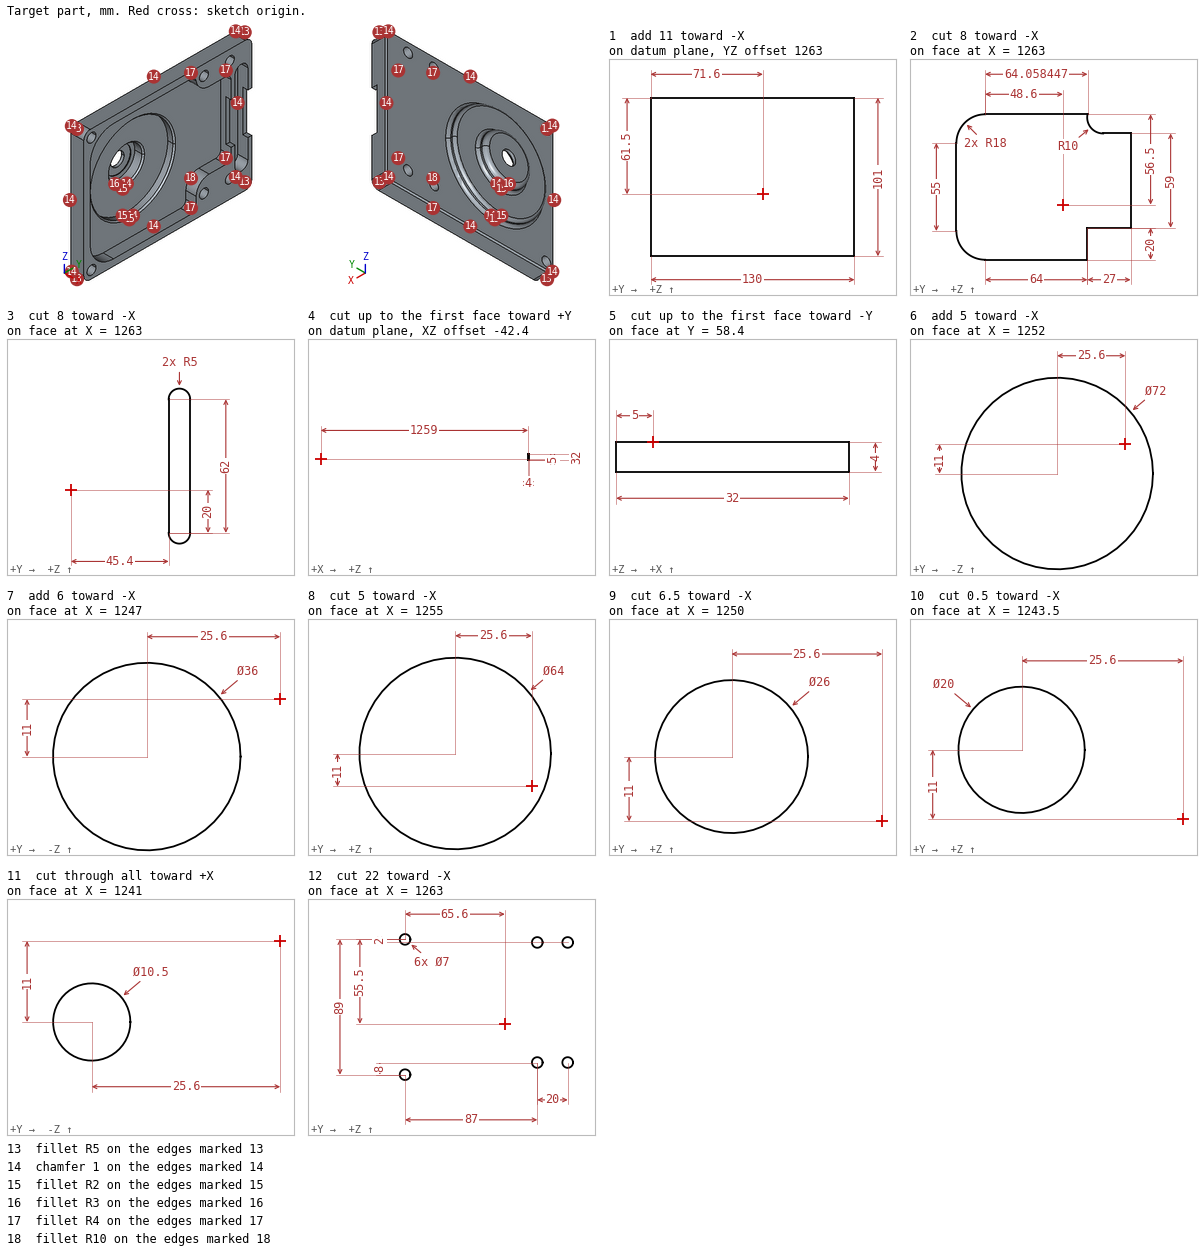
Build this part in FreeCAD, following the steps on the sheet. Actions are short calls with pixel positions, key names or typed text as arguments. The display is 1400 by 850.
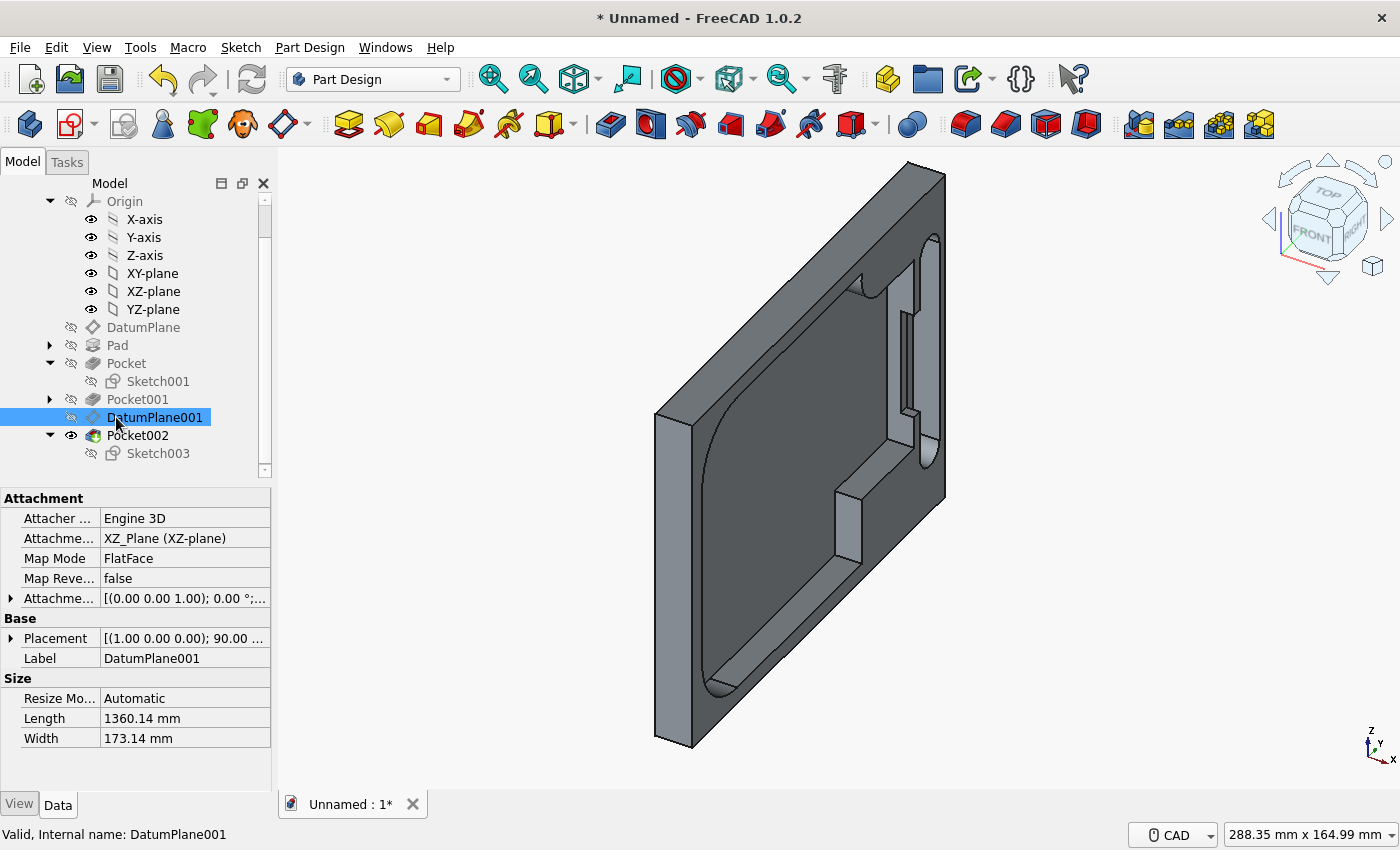
key(4)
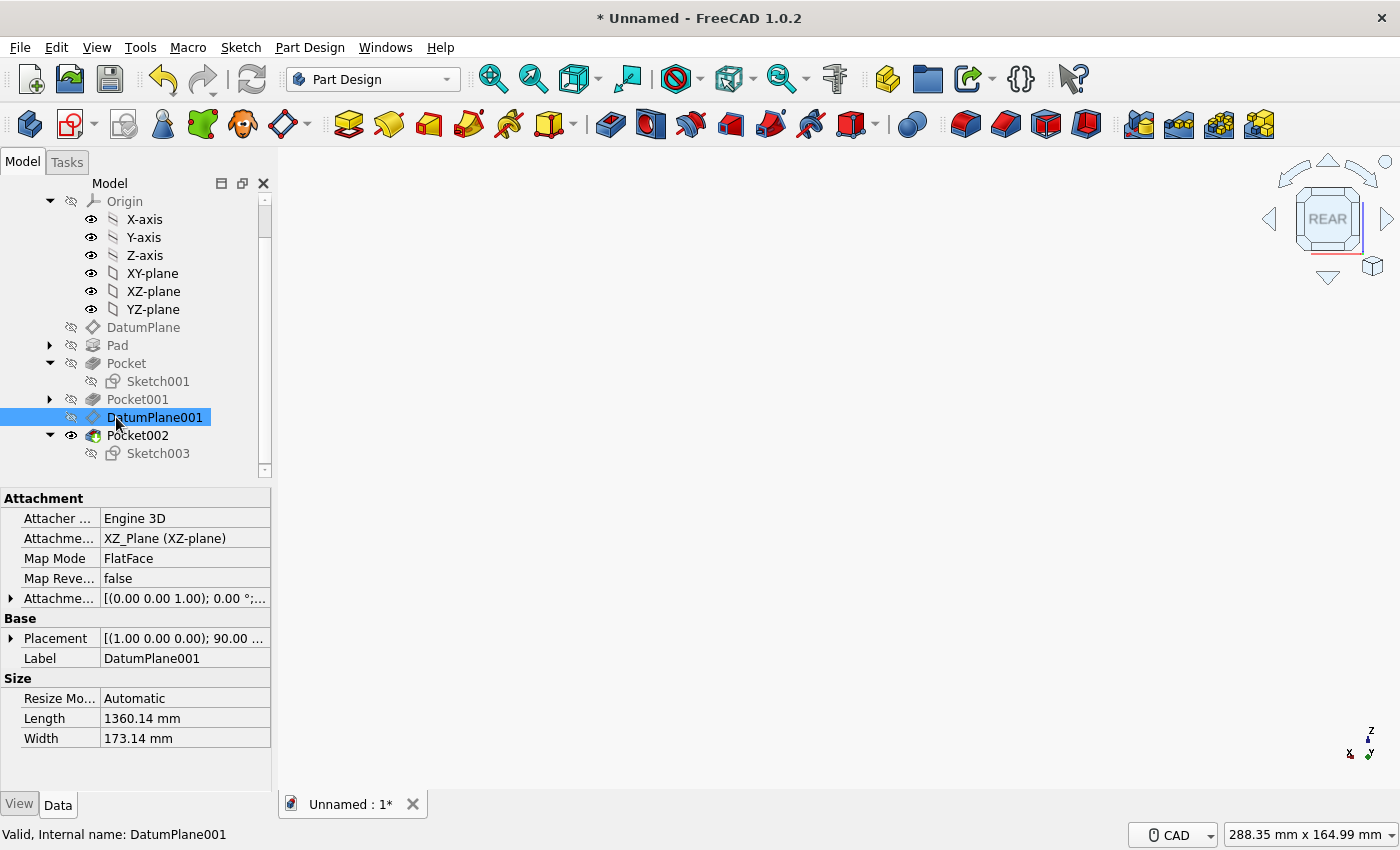
key(v)
key(f)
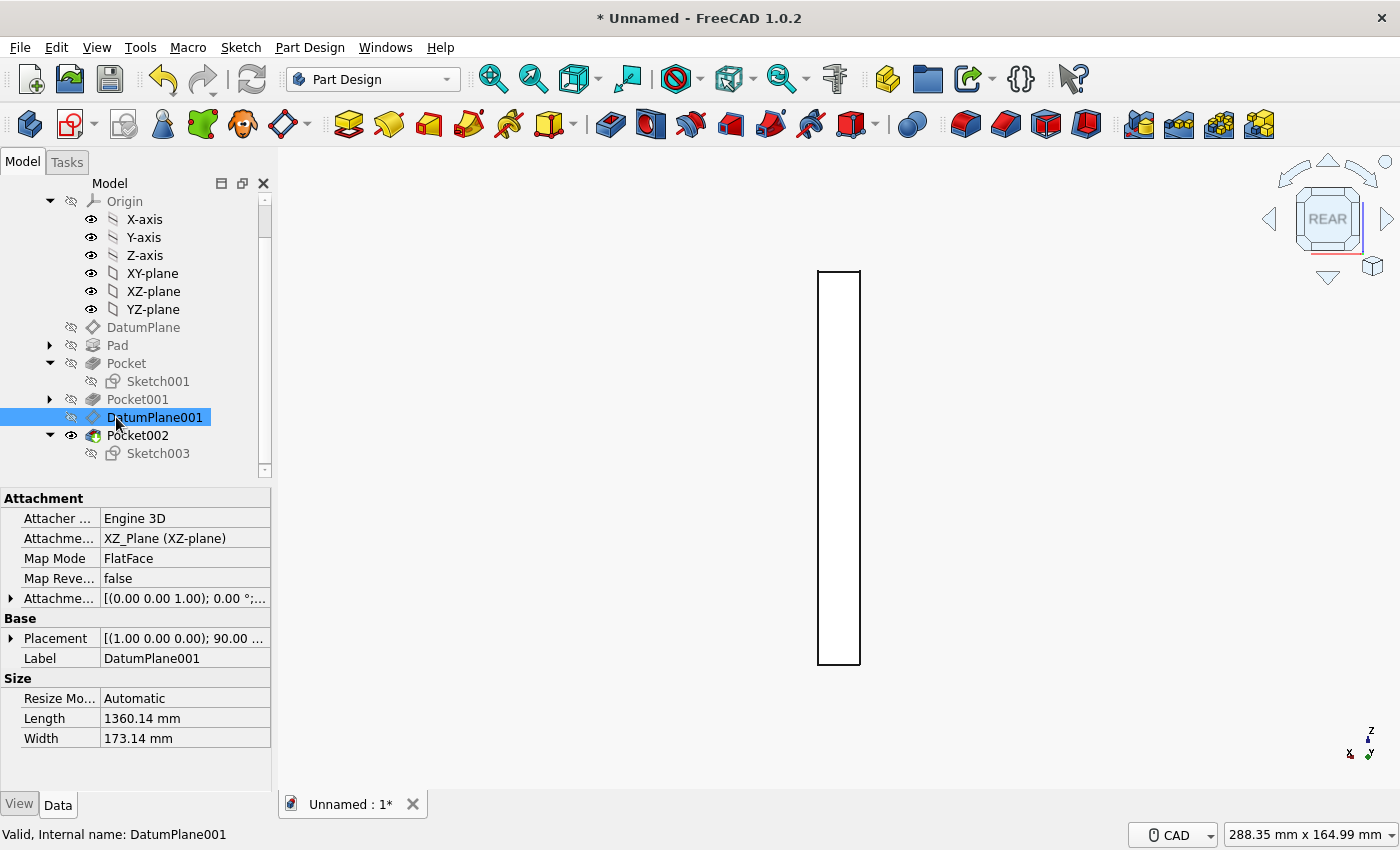
click(839, 299)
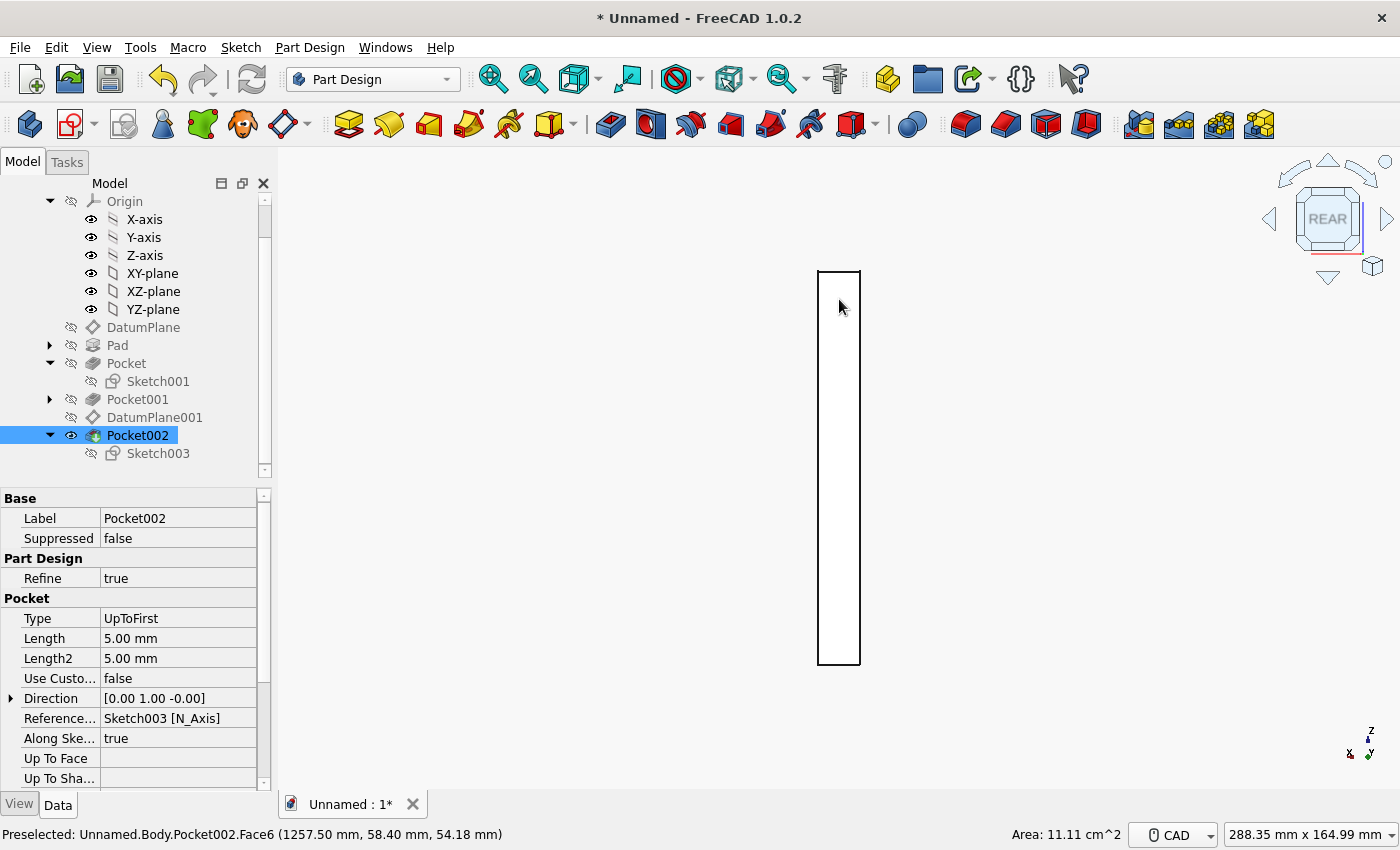
click(70, 124)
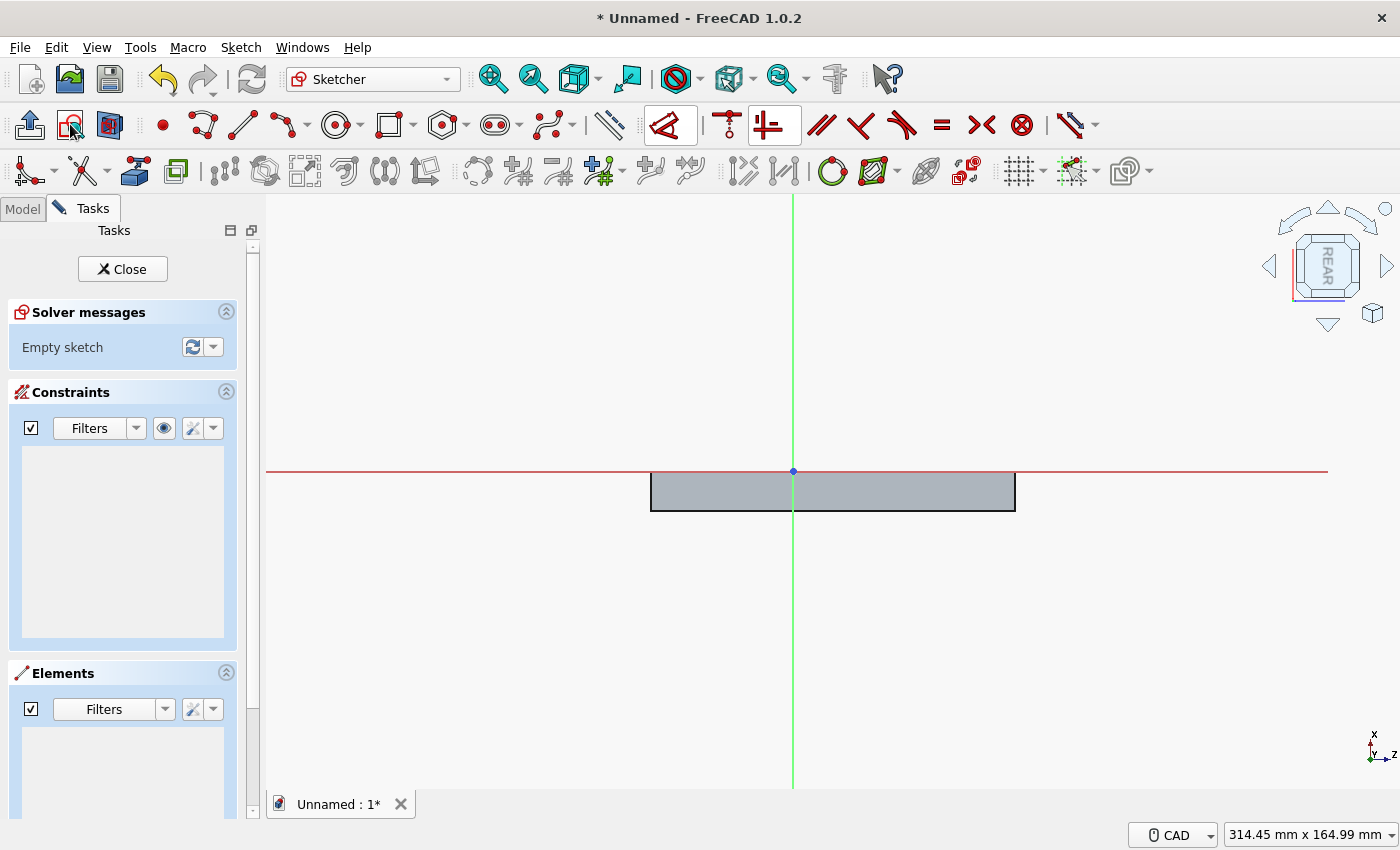
scroll(847, 476, up, 9)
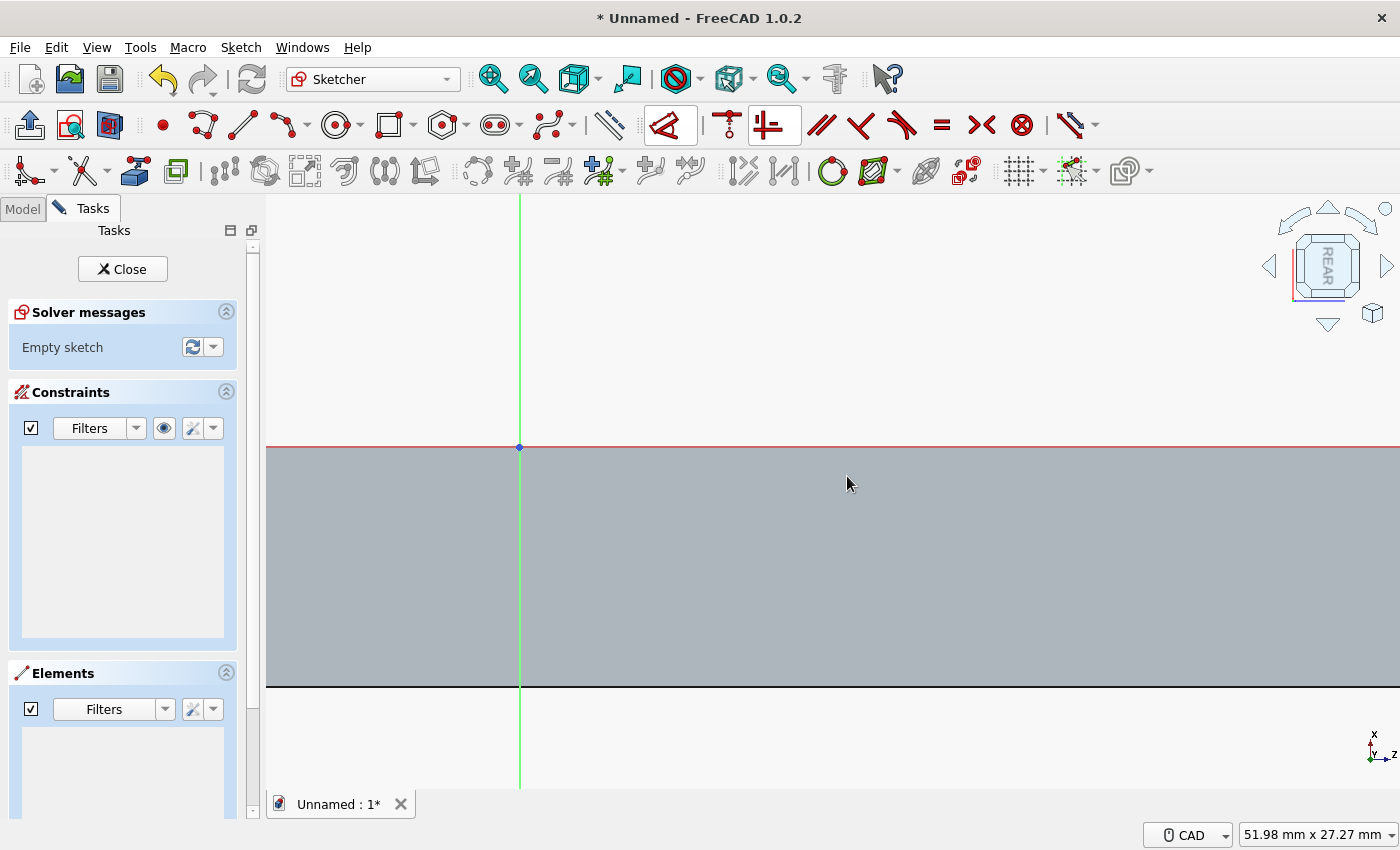
key(g)
key(r)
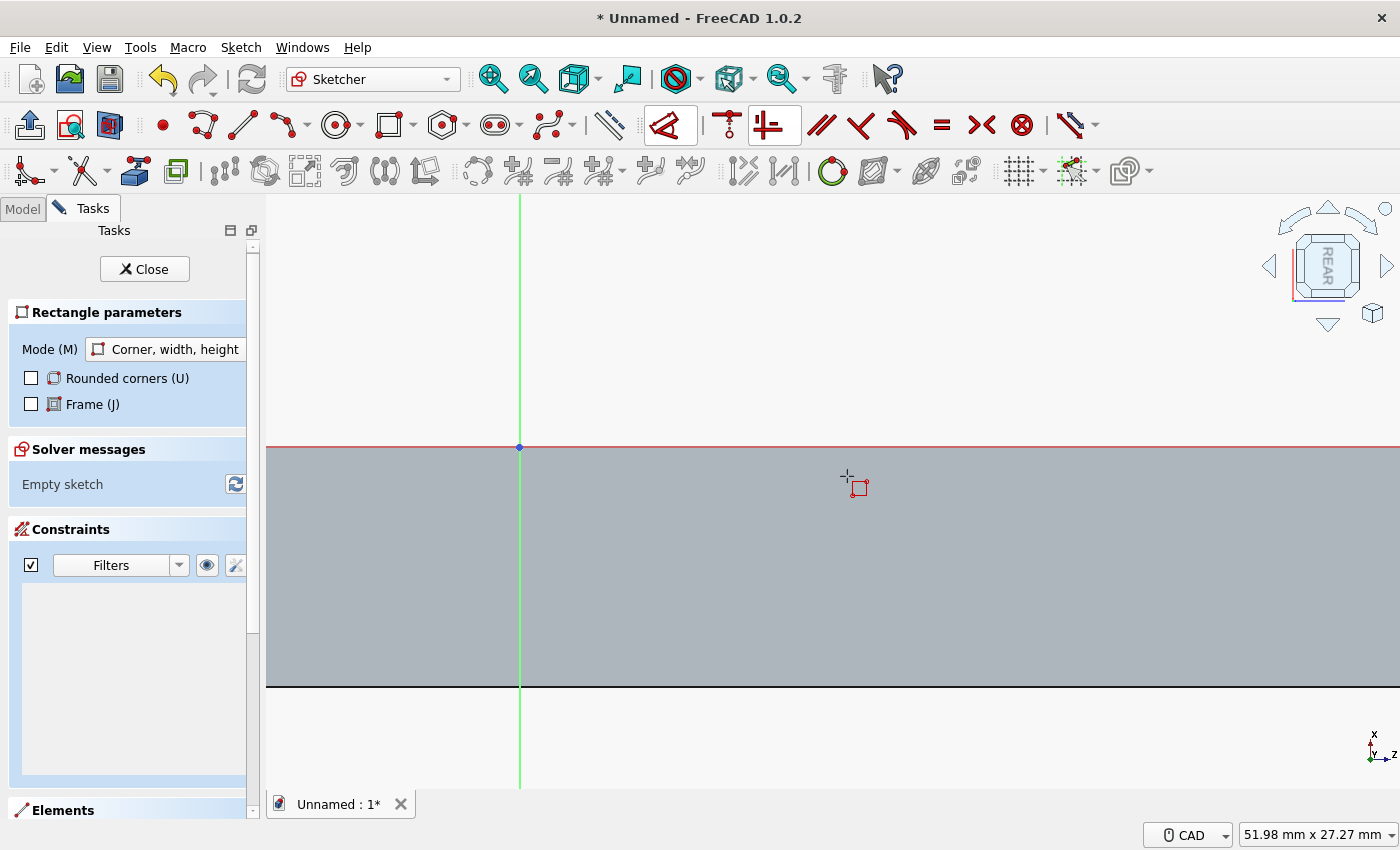
click(411, 447)
move(1109, 535)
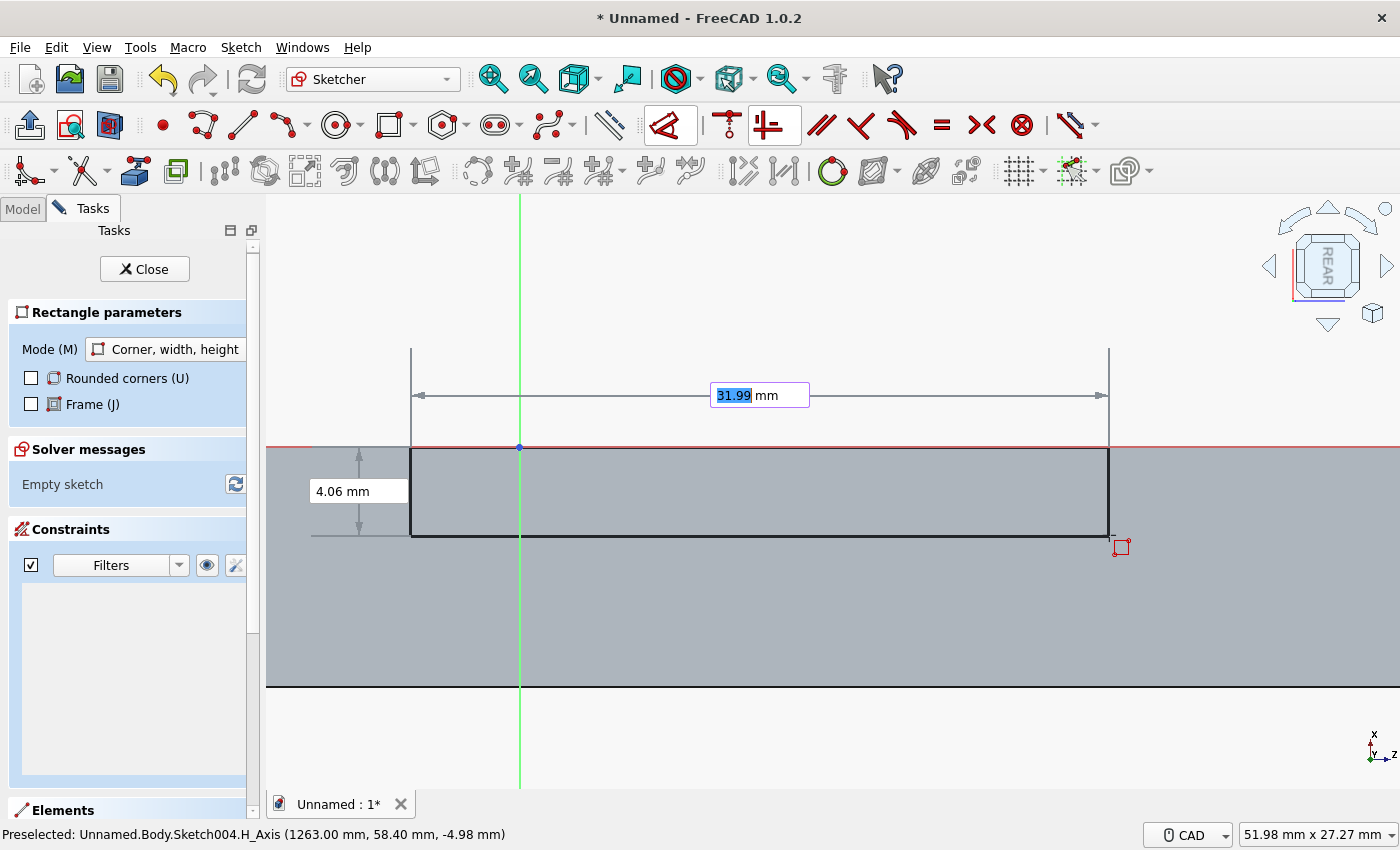
text(32)
key(Tab)
text(4)
key(Return)
key(Escape)